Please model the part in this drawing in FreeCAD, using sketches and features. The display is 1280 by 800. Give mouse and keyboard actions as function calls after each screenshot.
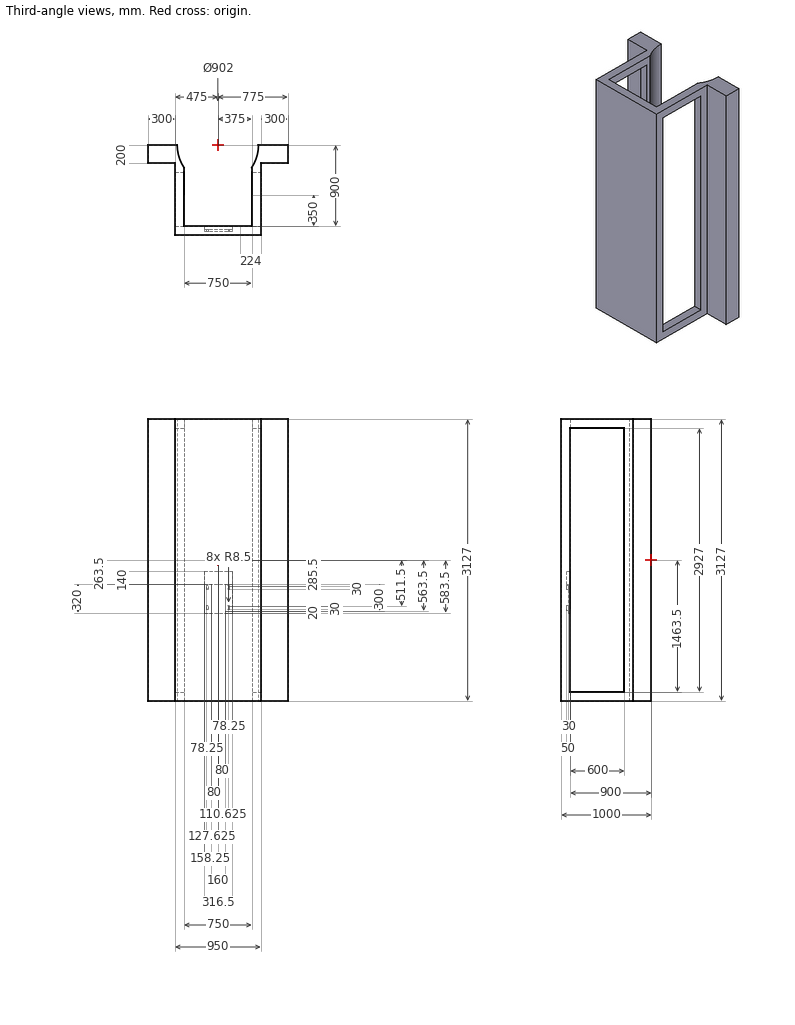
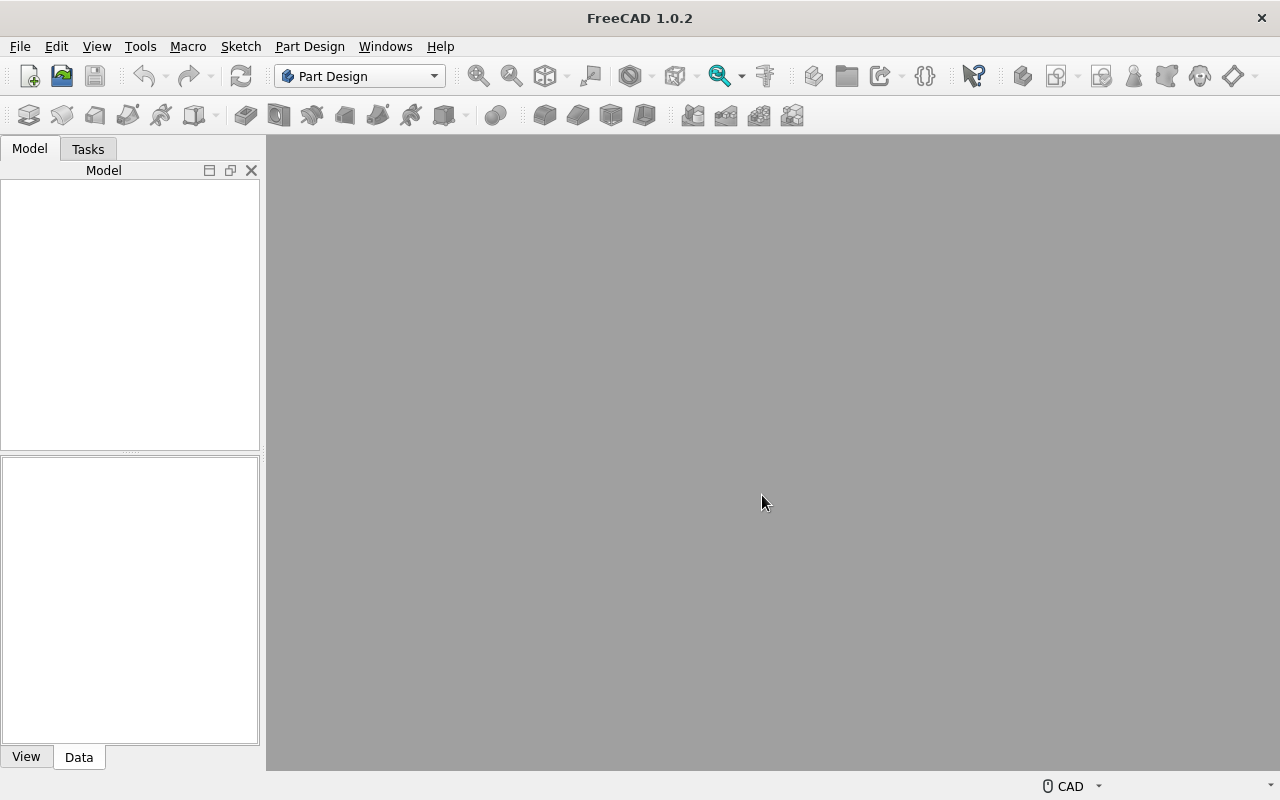
click(29, 76)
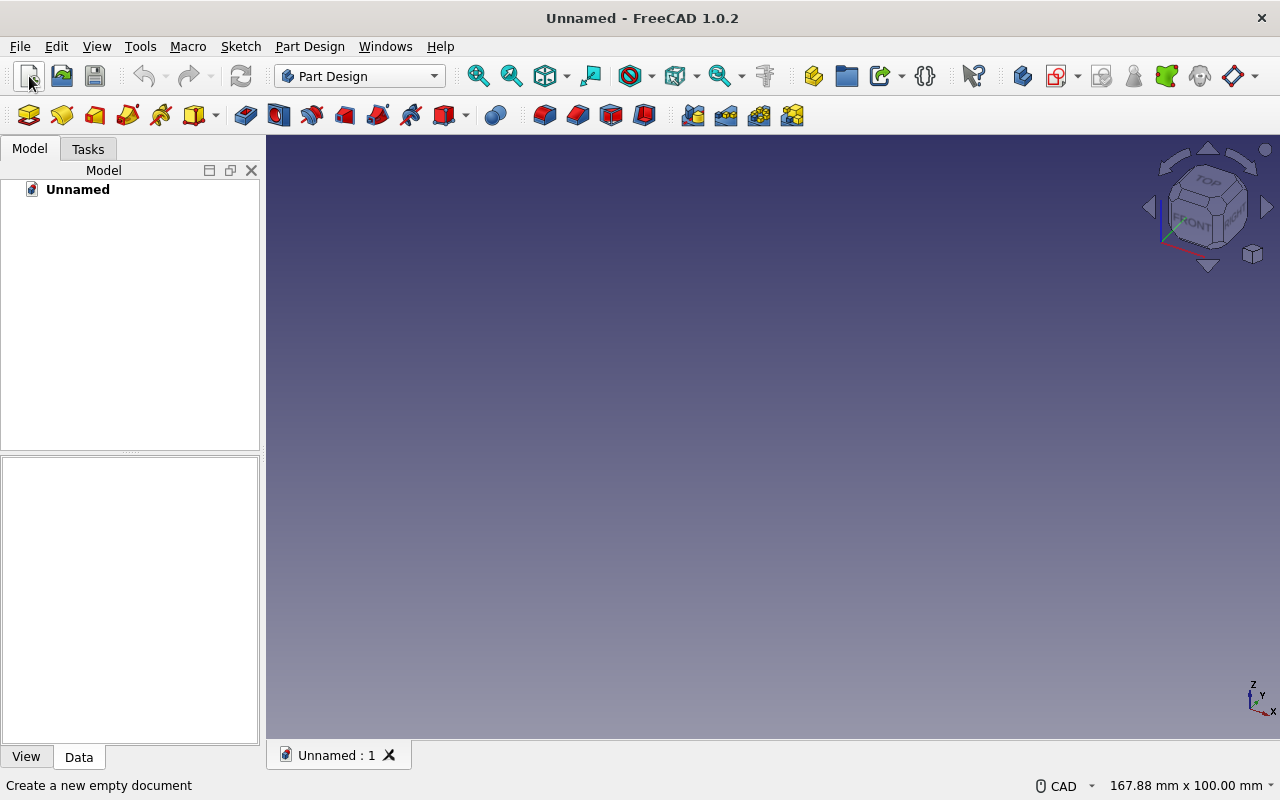
click(1056, 76)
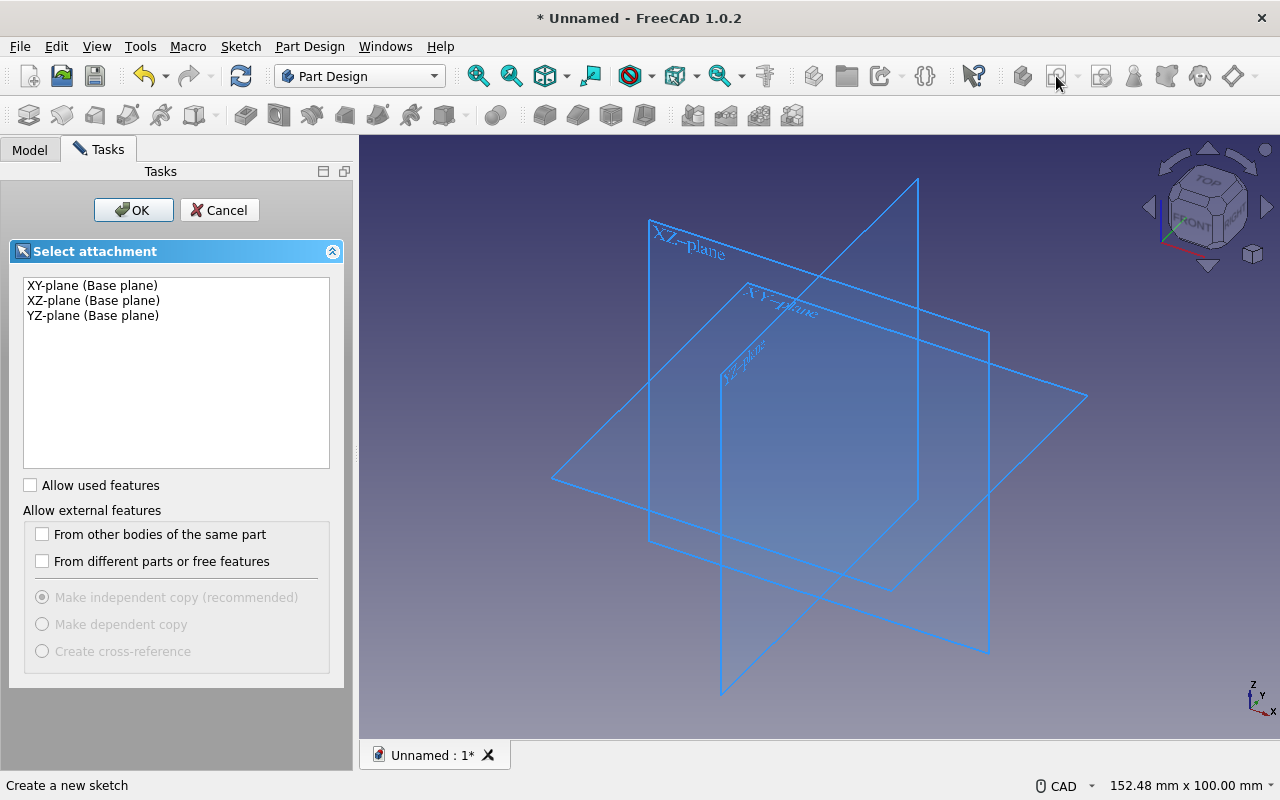
click(84, 300)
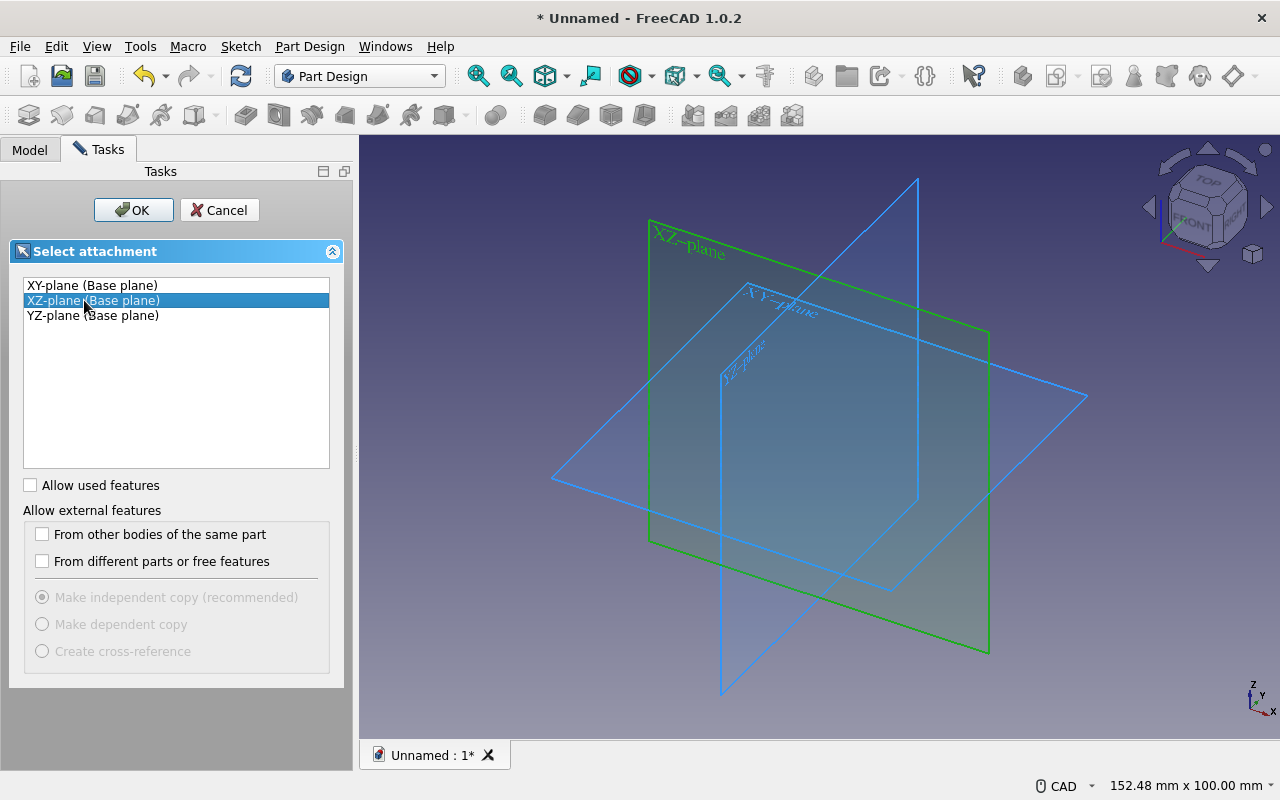
click(134, 210)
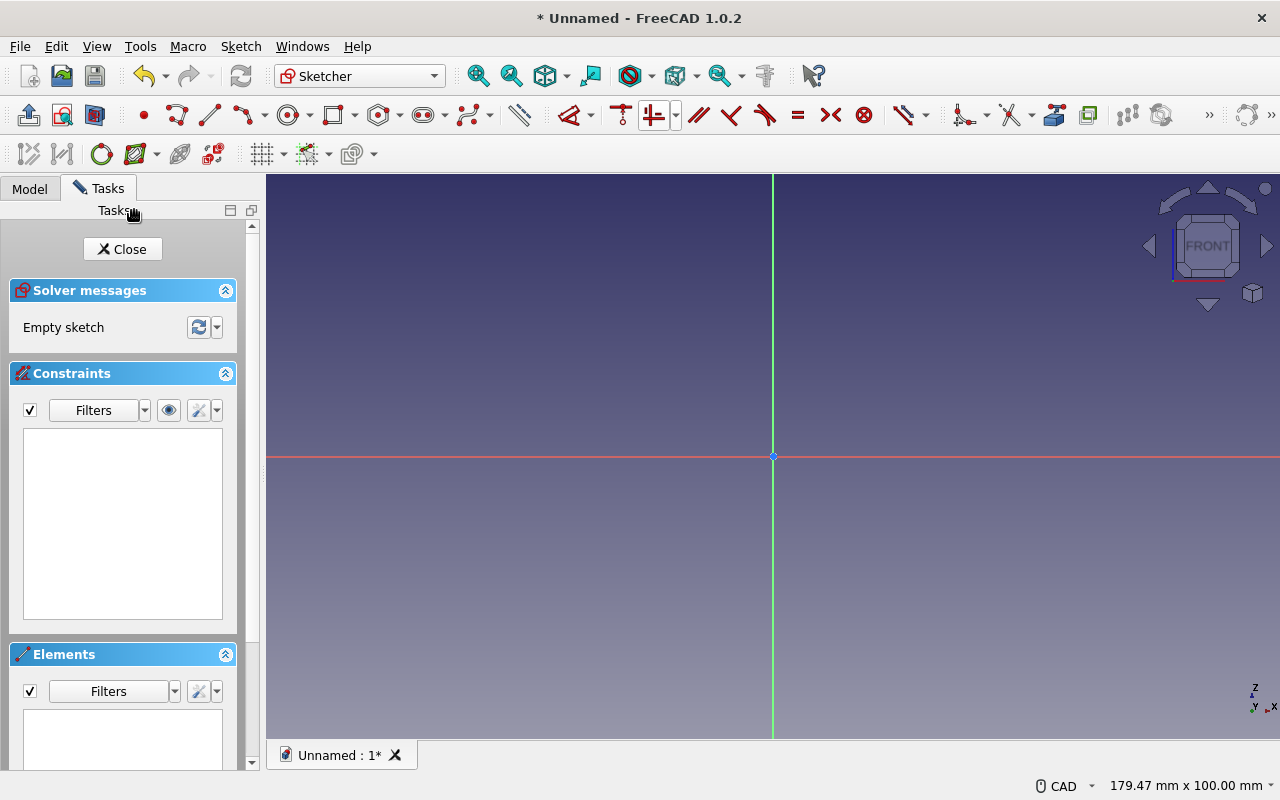
scroll(704, 456, down, 15)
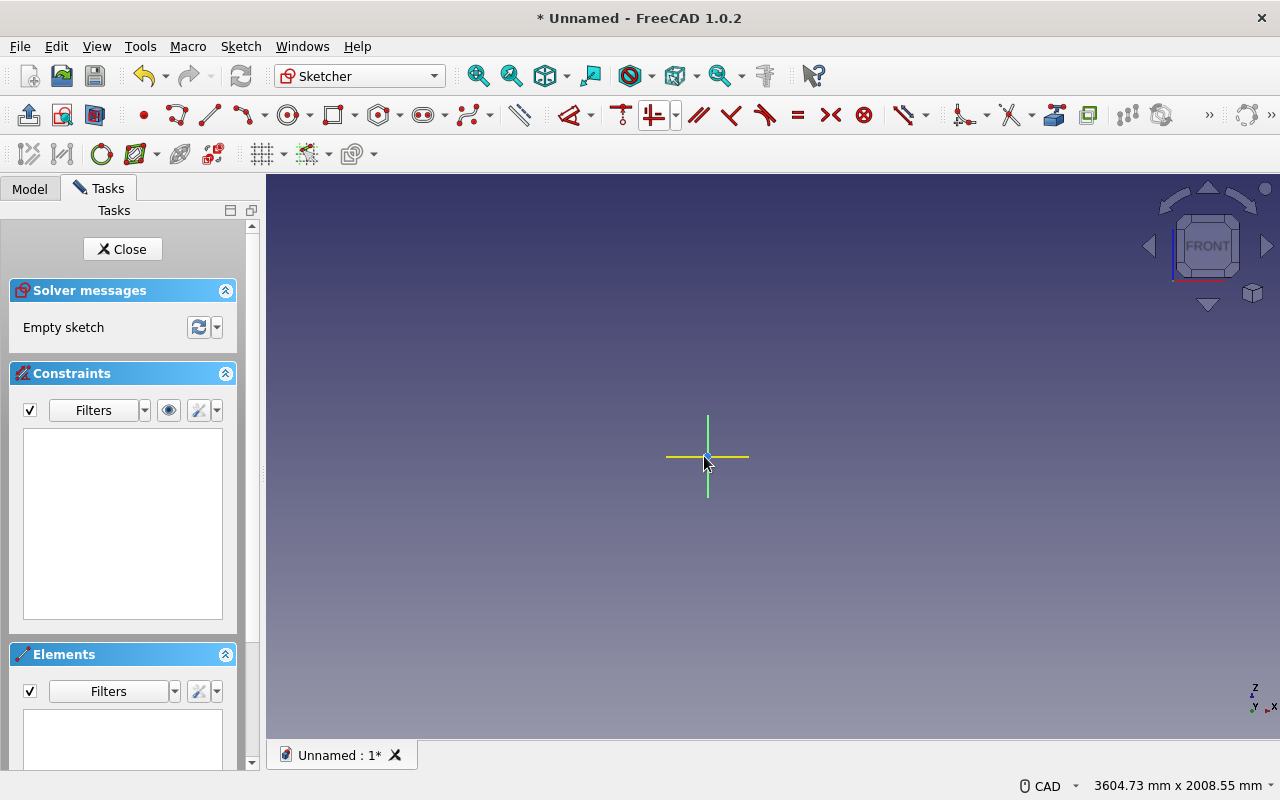
scroll(702, 456, down, 4)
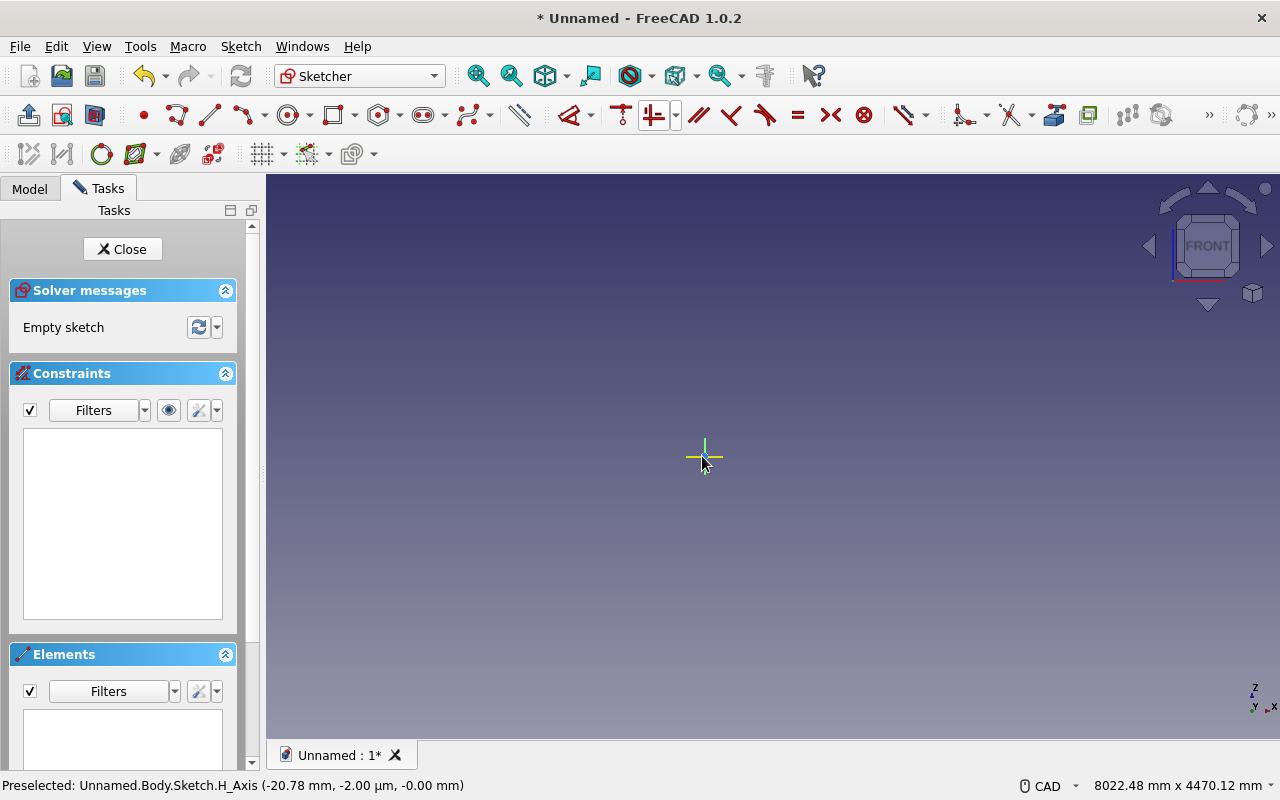
click(354, 116)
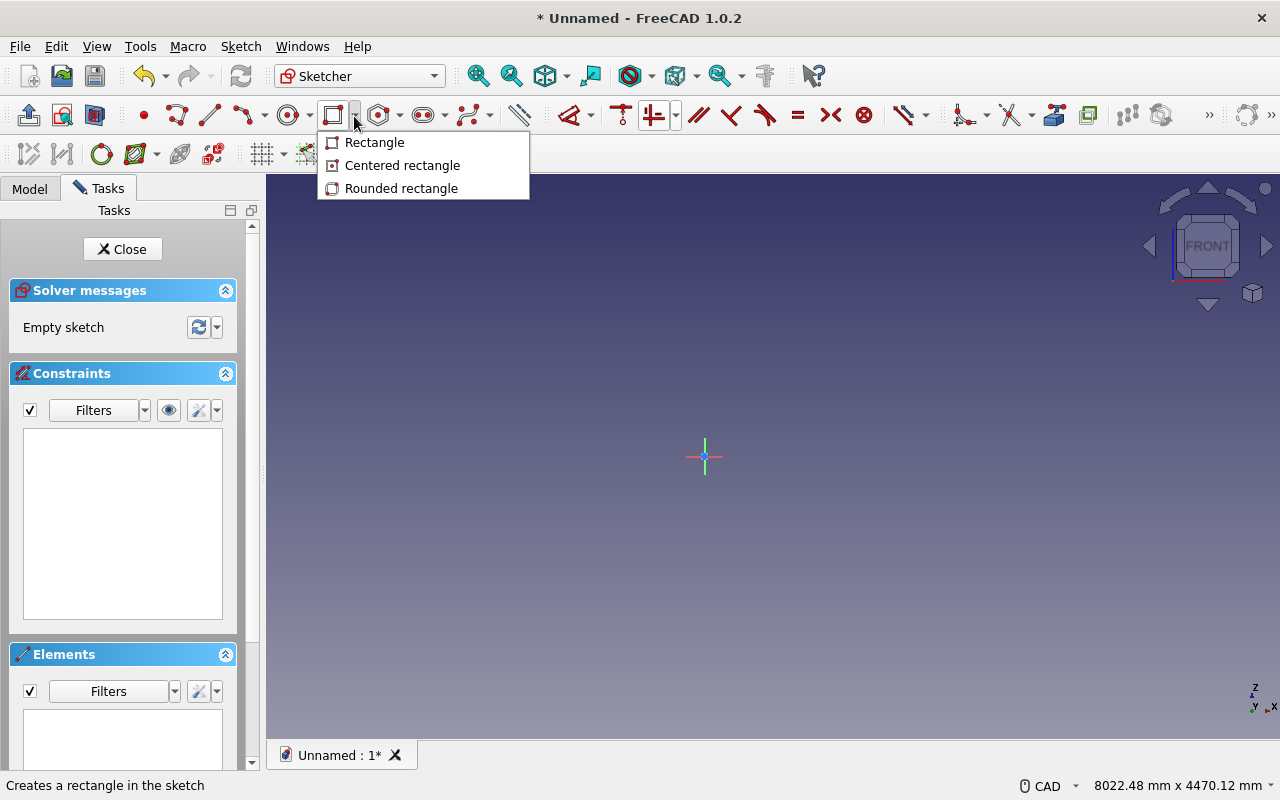
click(424, 166)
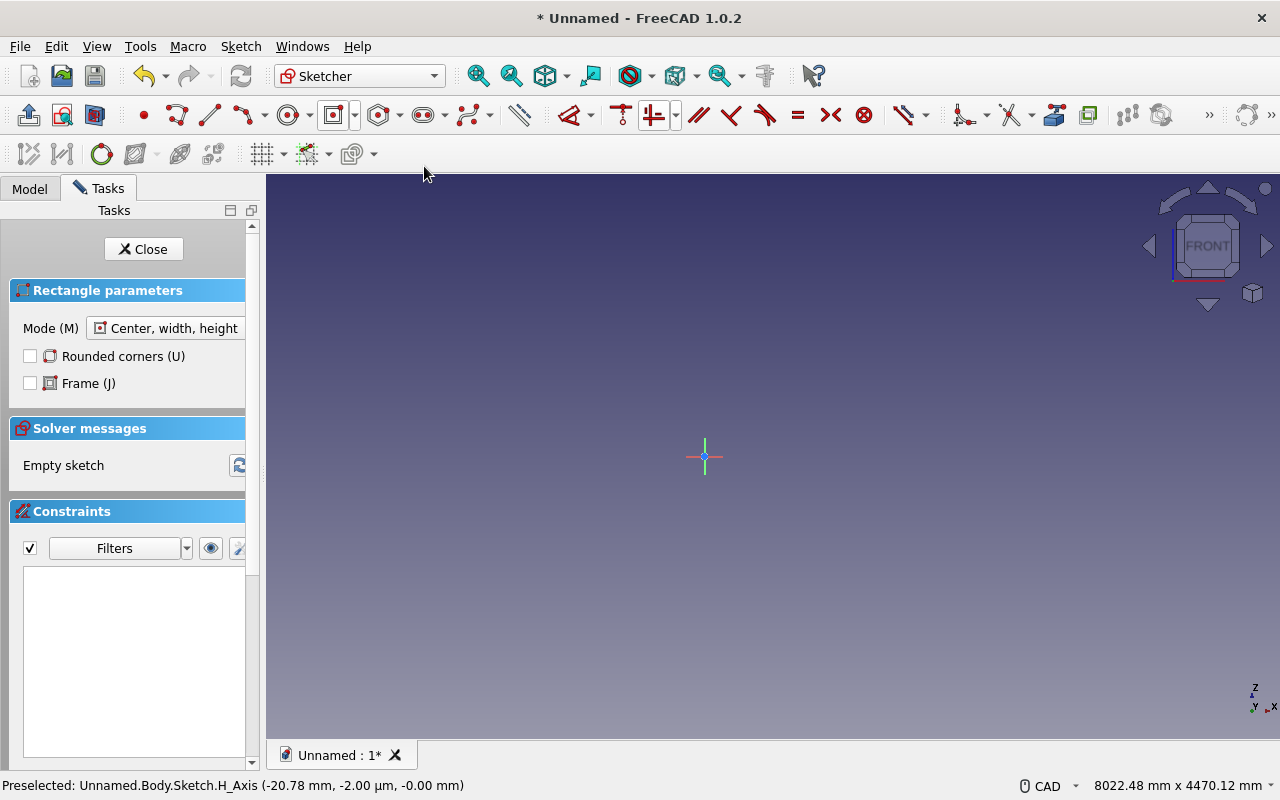
click(705, 456)
click(765, 259)
key(Escape)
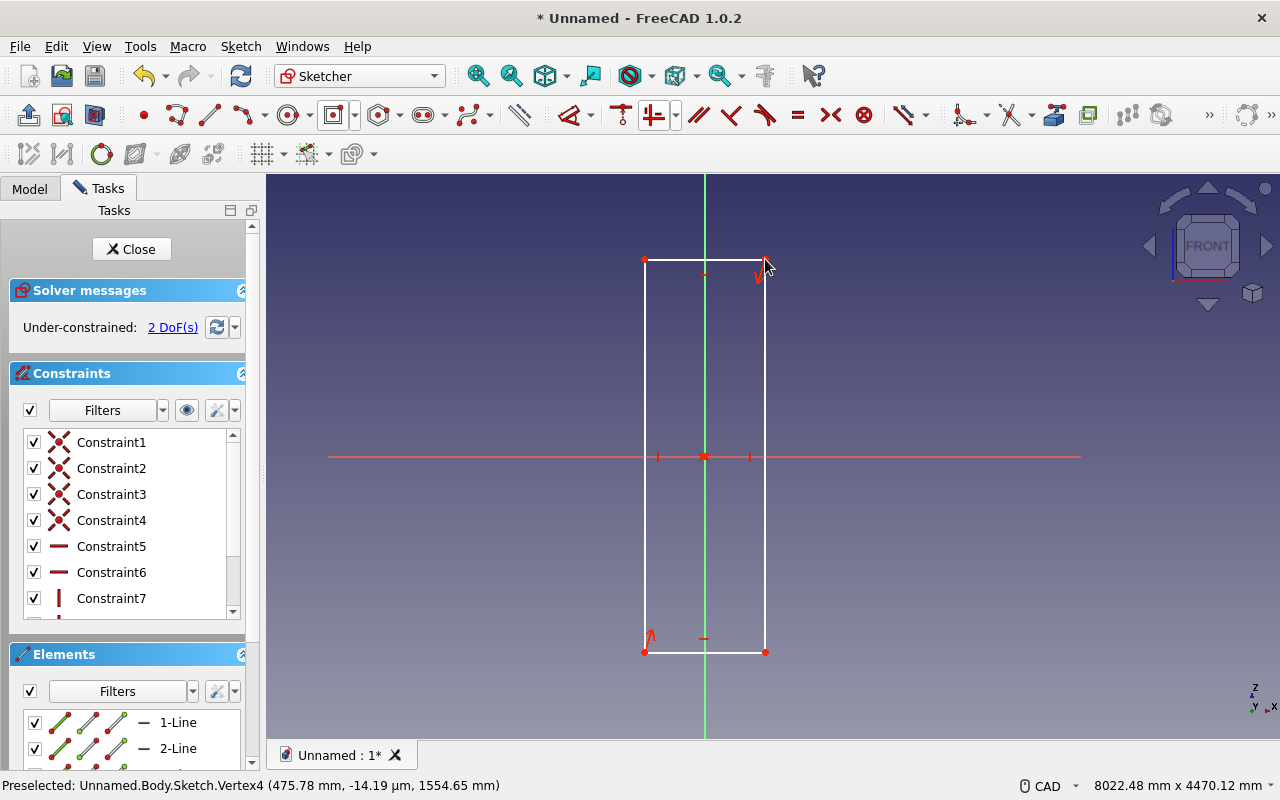
click(568, 116)